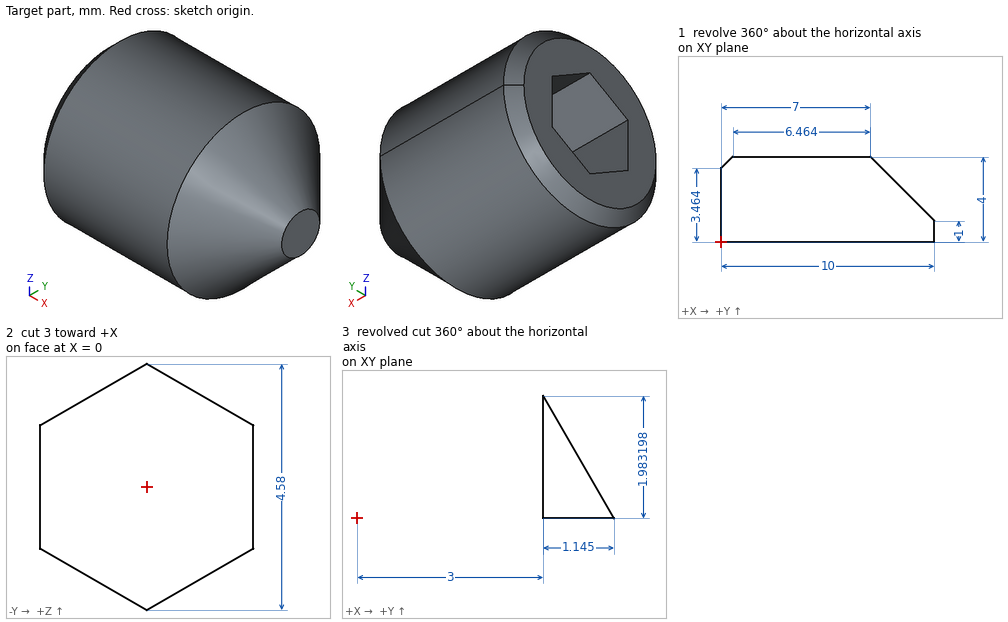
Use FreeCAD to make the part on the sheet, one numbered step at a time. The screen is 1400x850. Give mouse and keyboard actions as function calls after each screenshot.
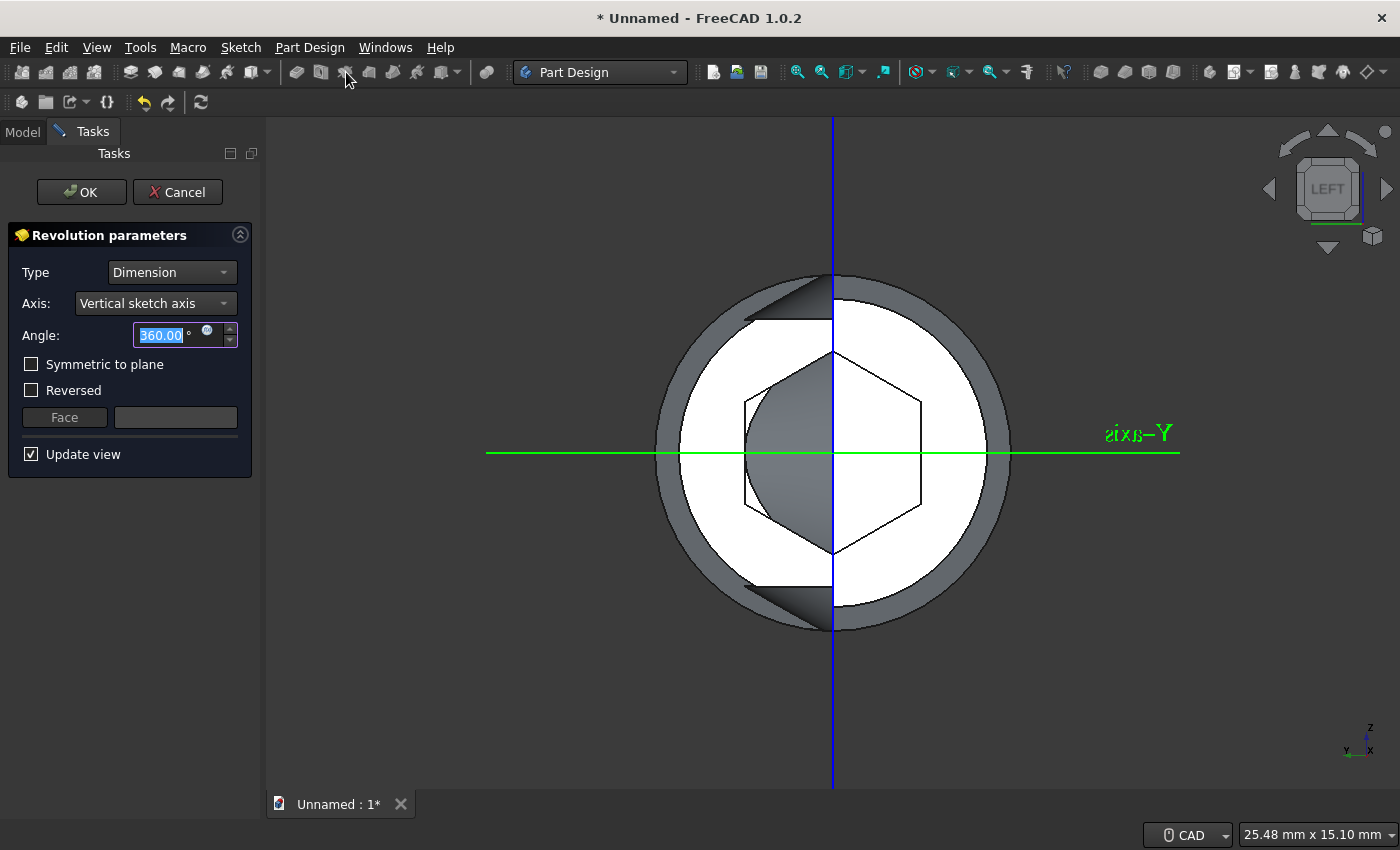
click(156, 304)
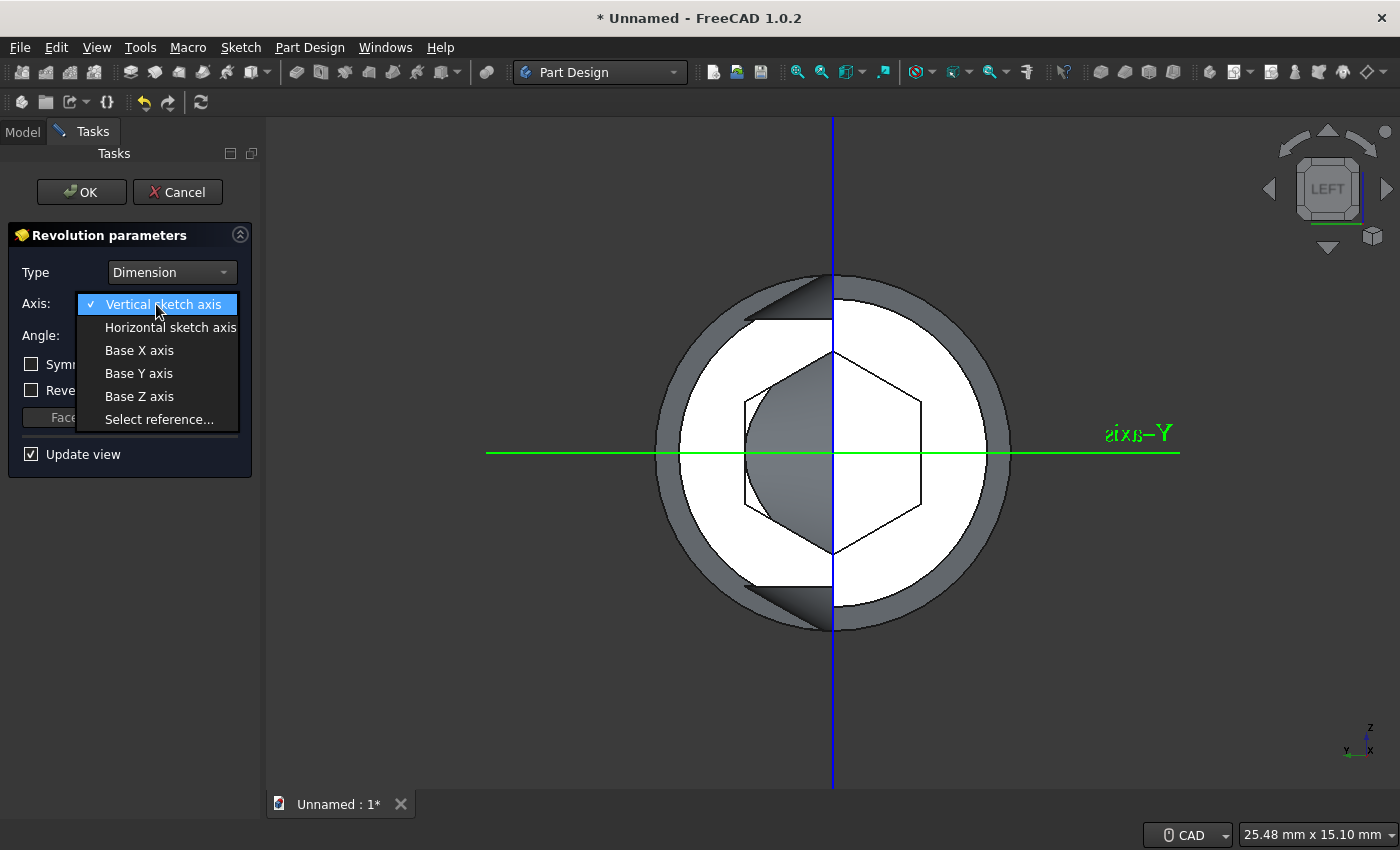
click(156, 328)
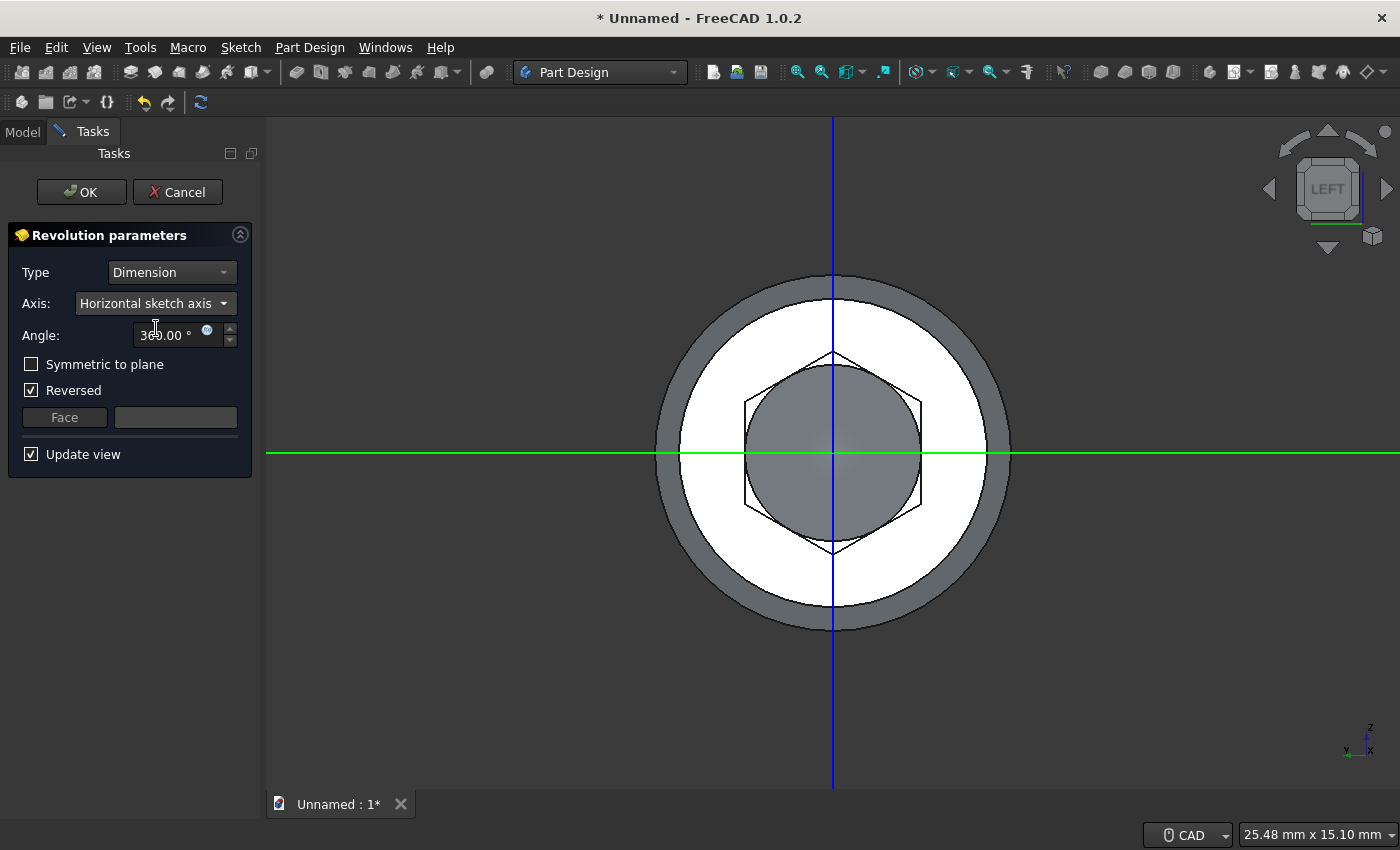
click(82, 192)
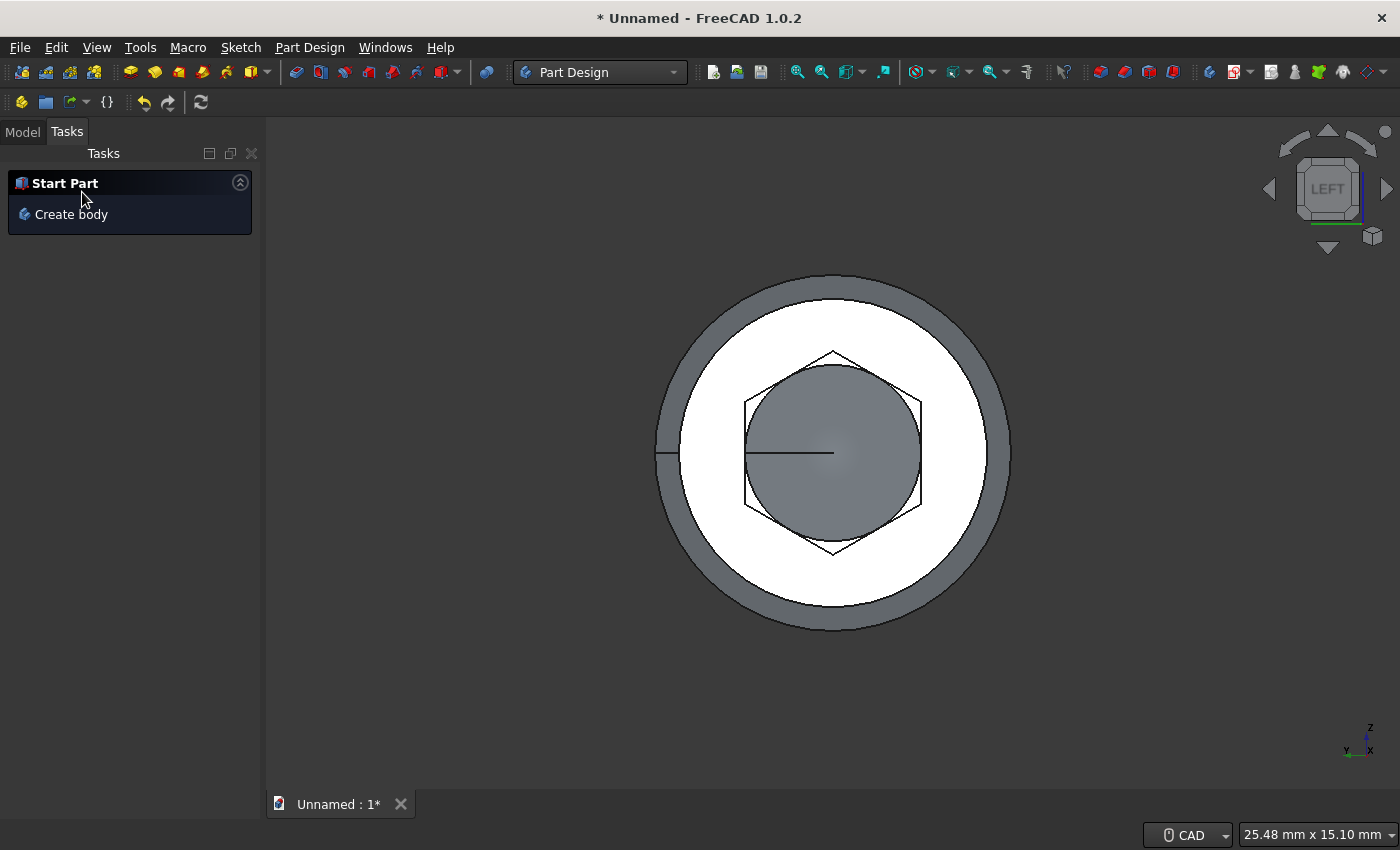
key(0)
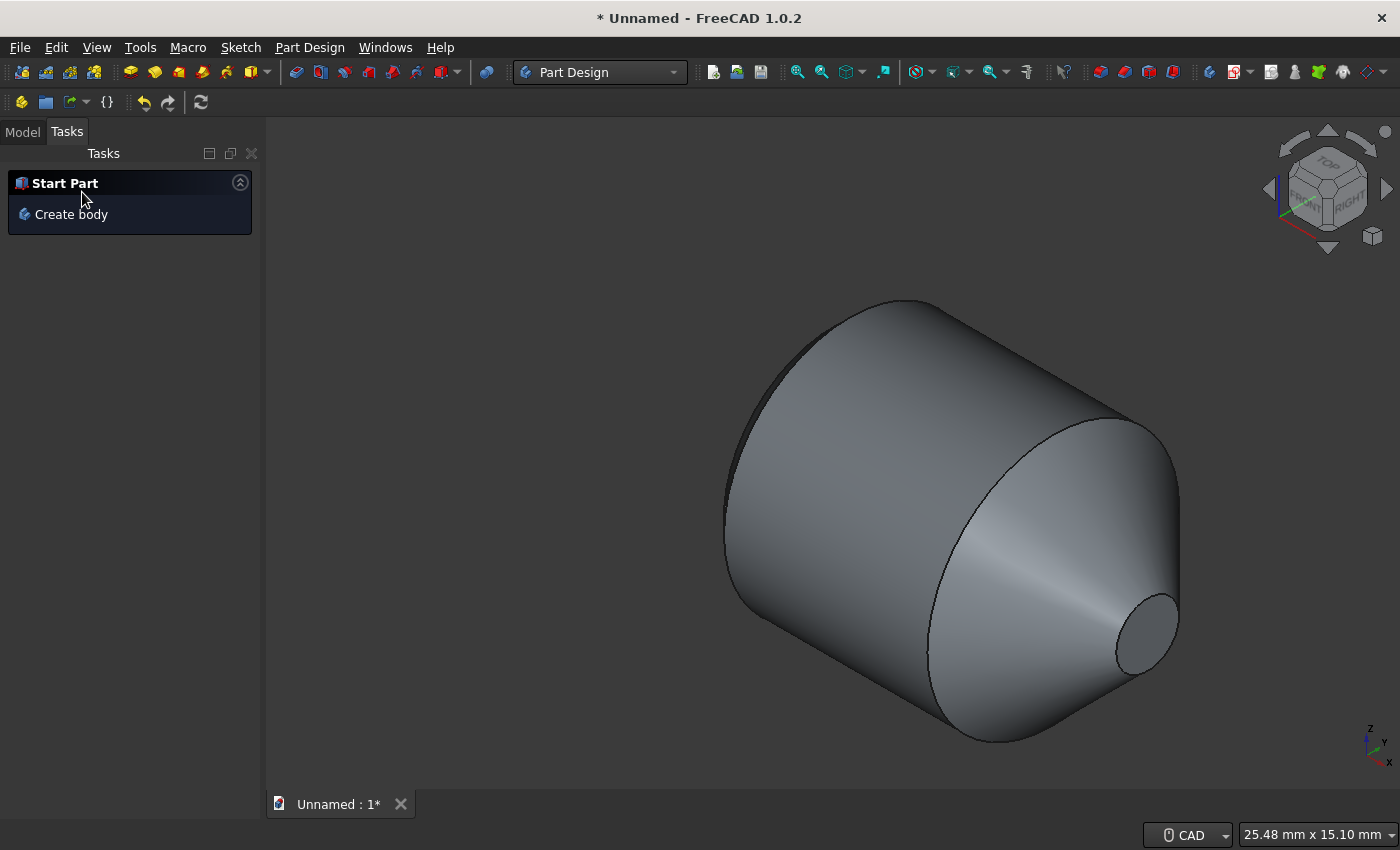
click(798, 72)